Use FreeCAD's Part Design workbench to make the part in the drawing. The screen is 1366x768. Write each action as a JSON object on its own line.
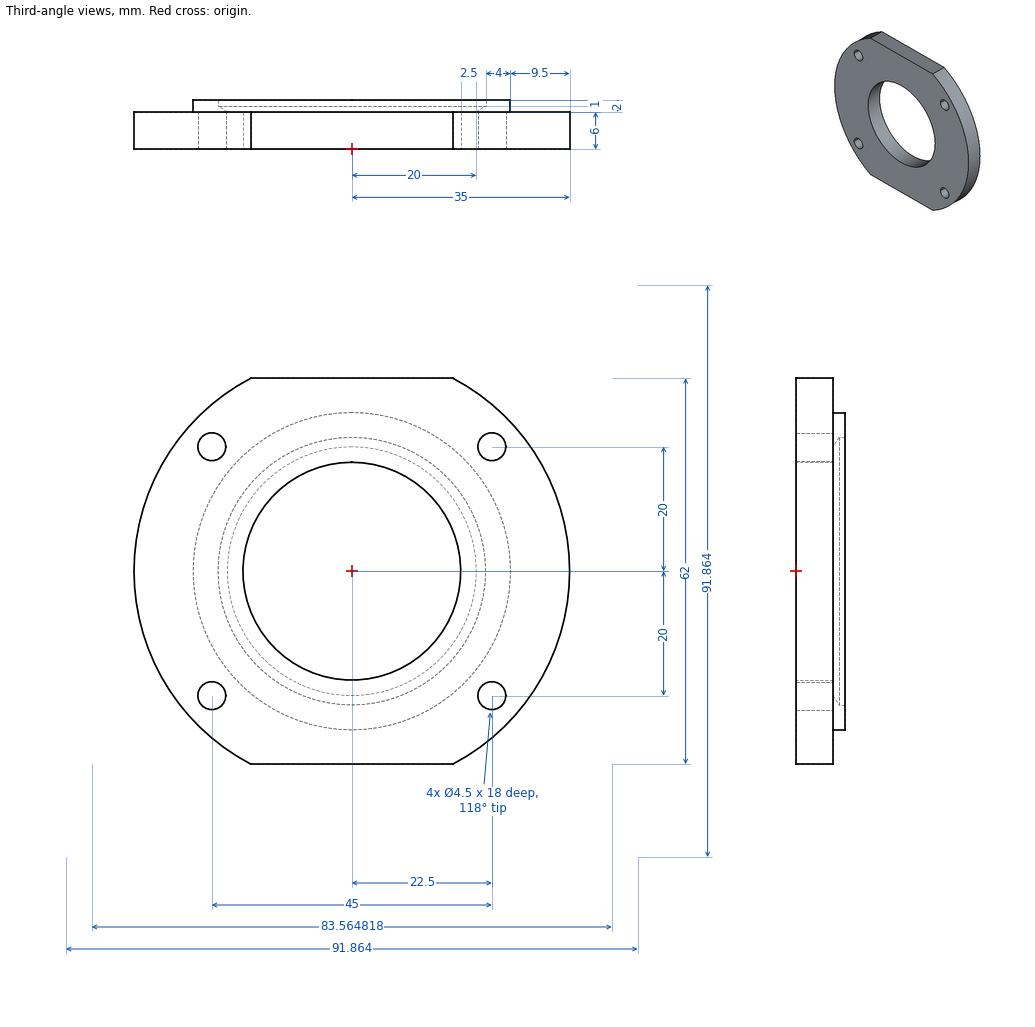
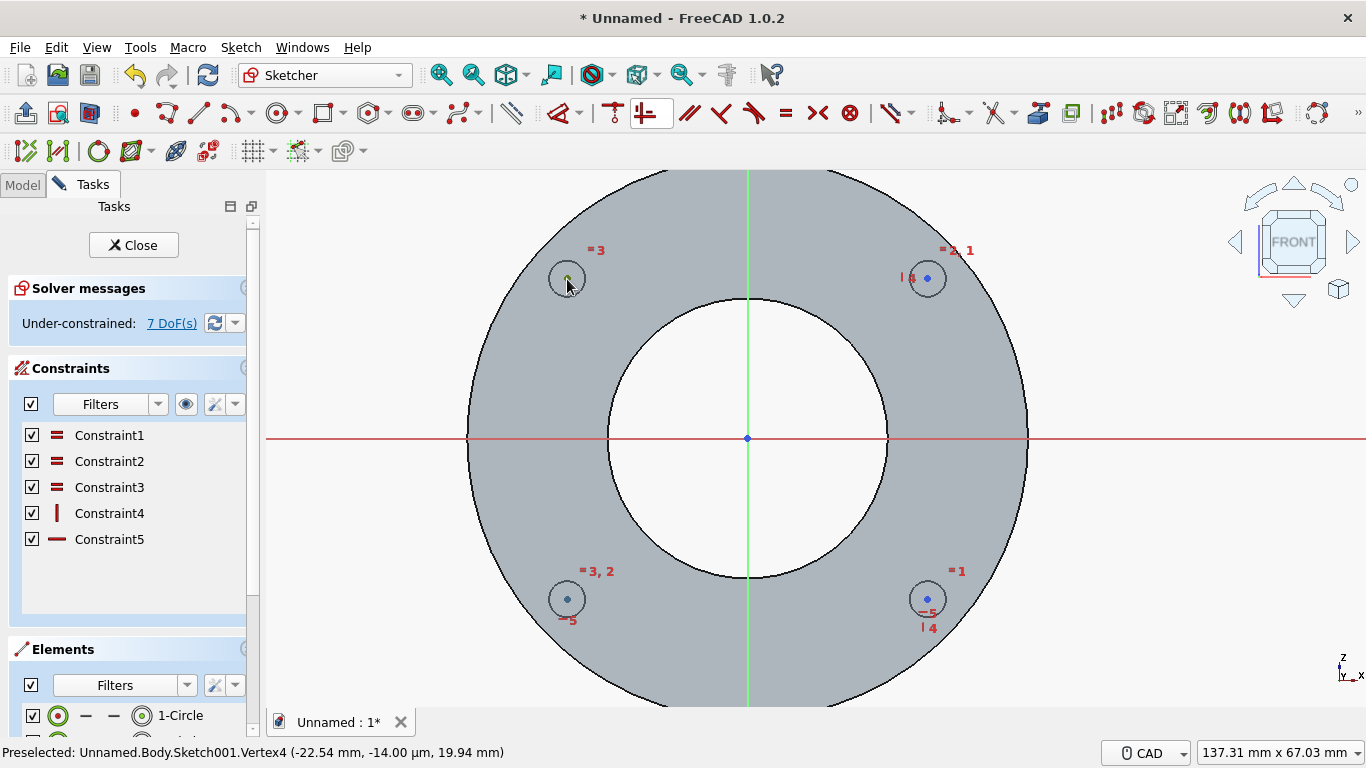
{"action": "key", "text": "v"}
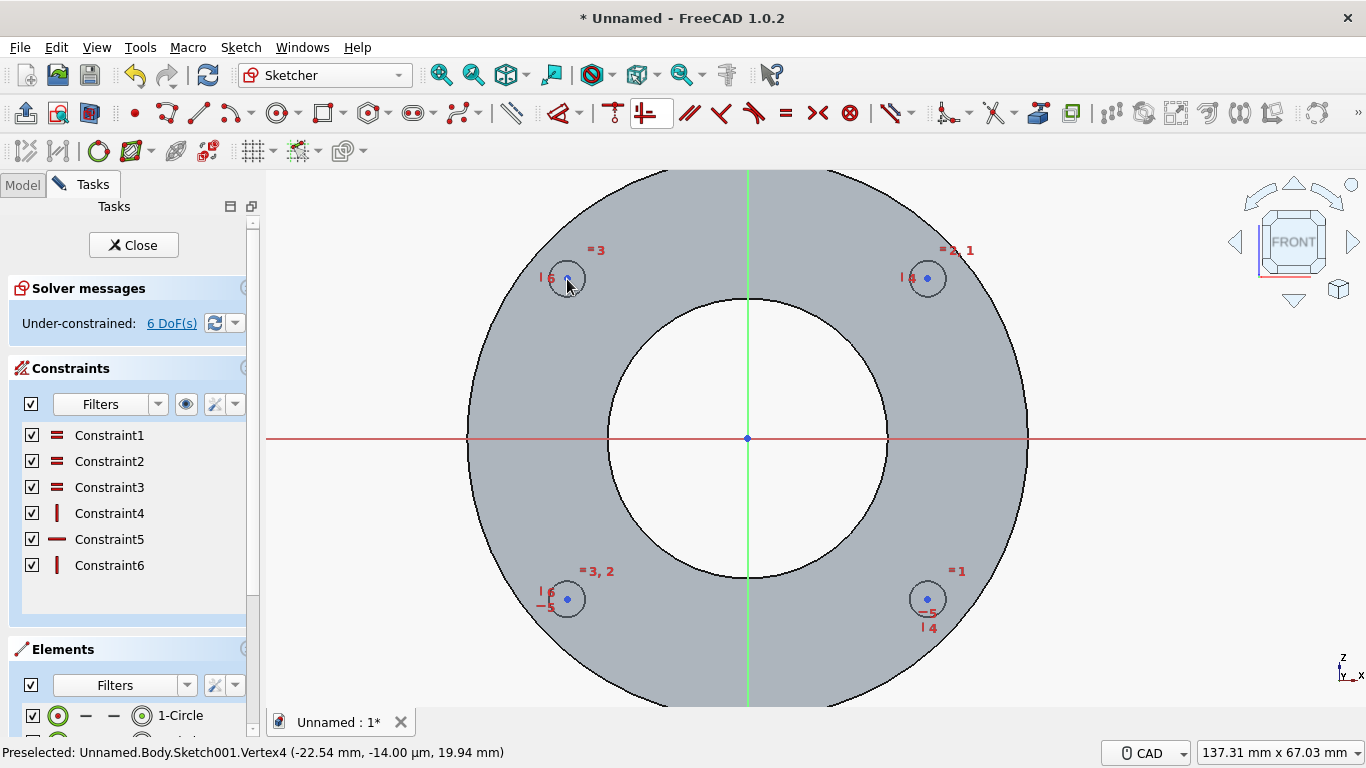
{"action": "left_click", "coordinate": [928, 279]}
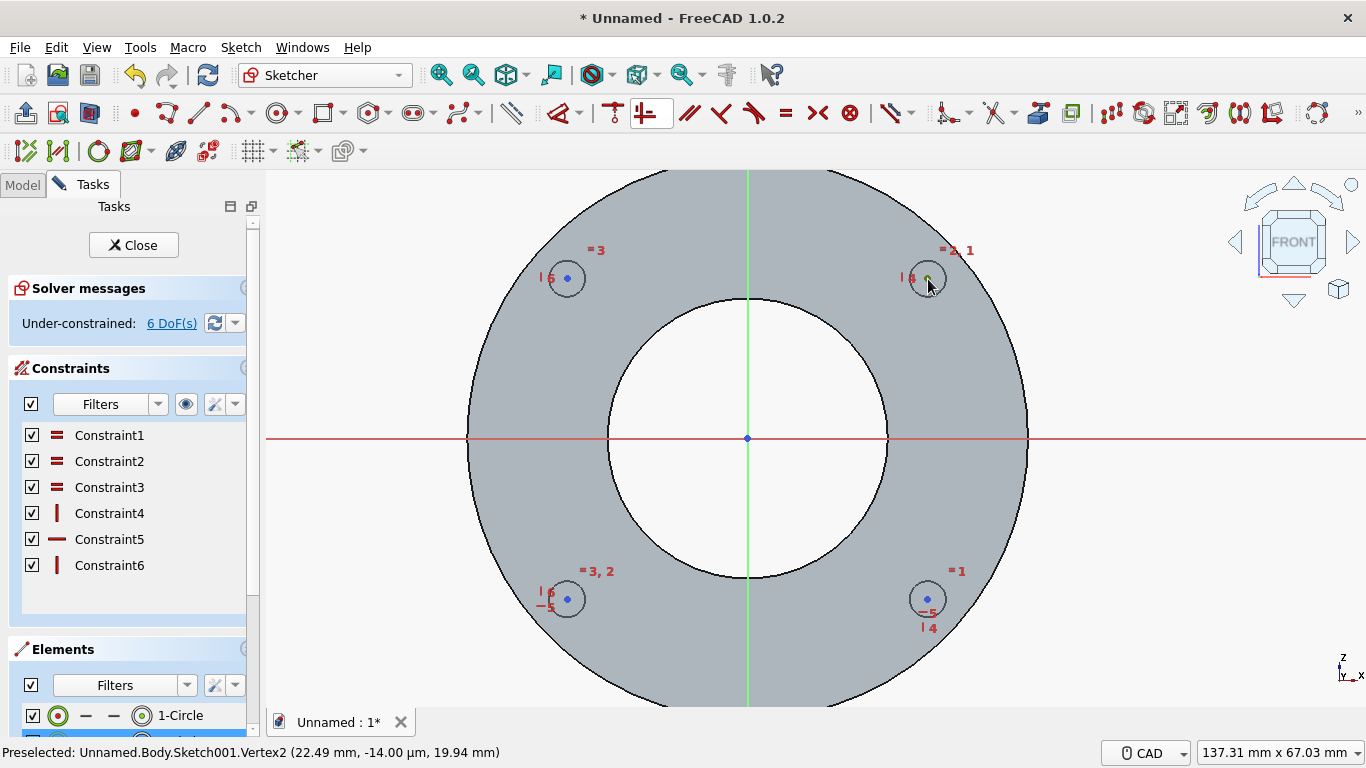
{"action": "left_click", "coordinate": [567, 279]}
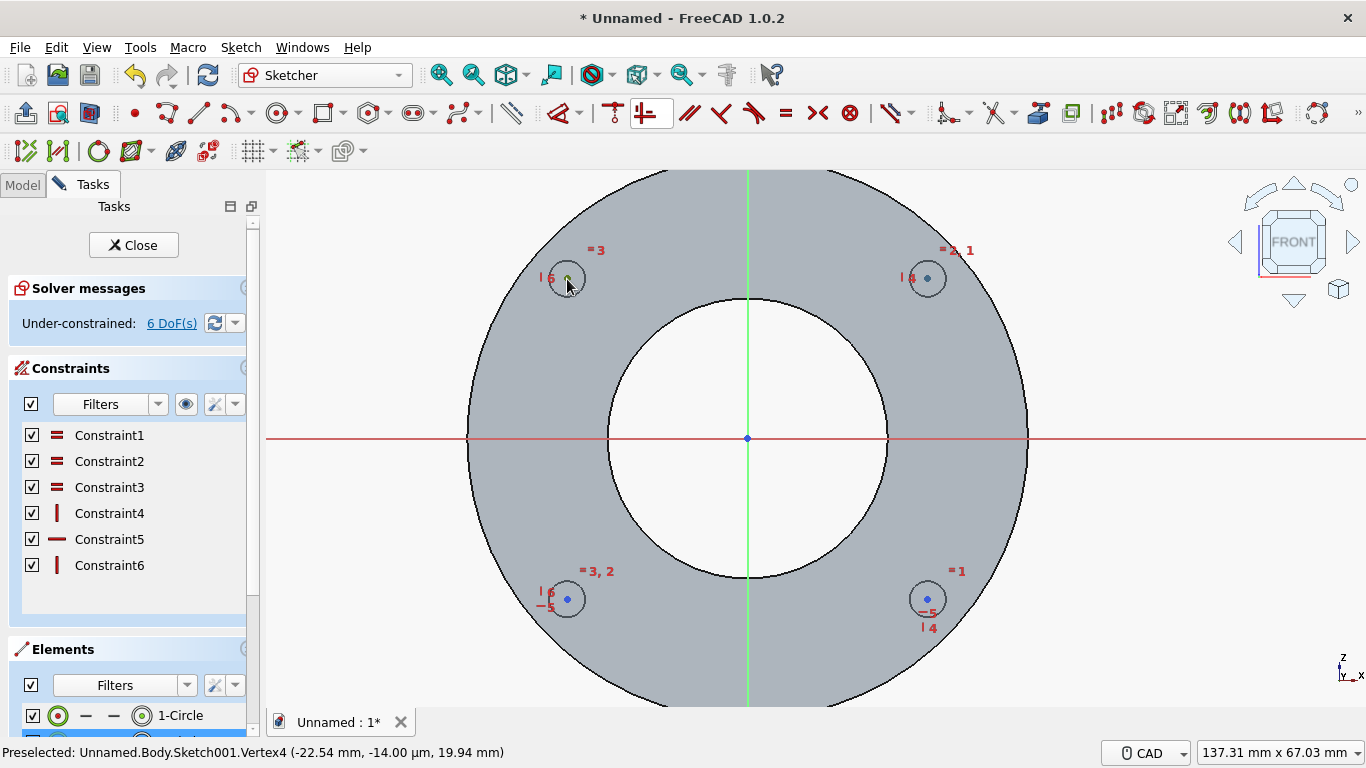
{"action": "key", "text": "h"}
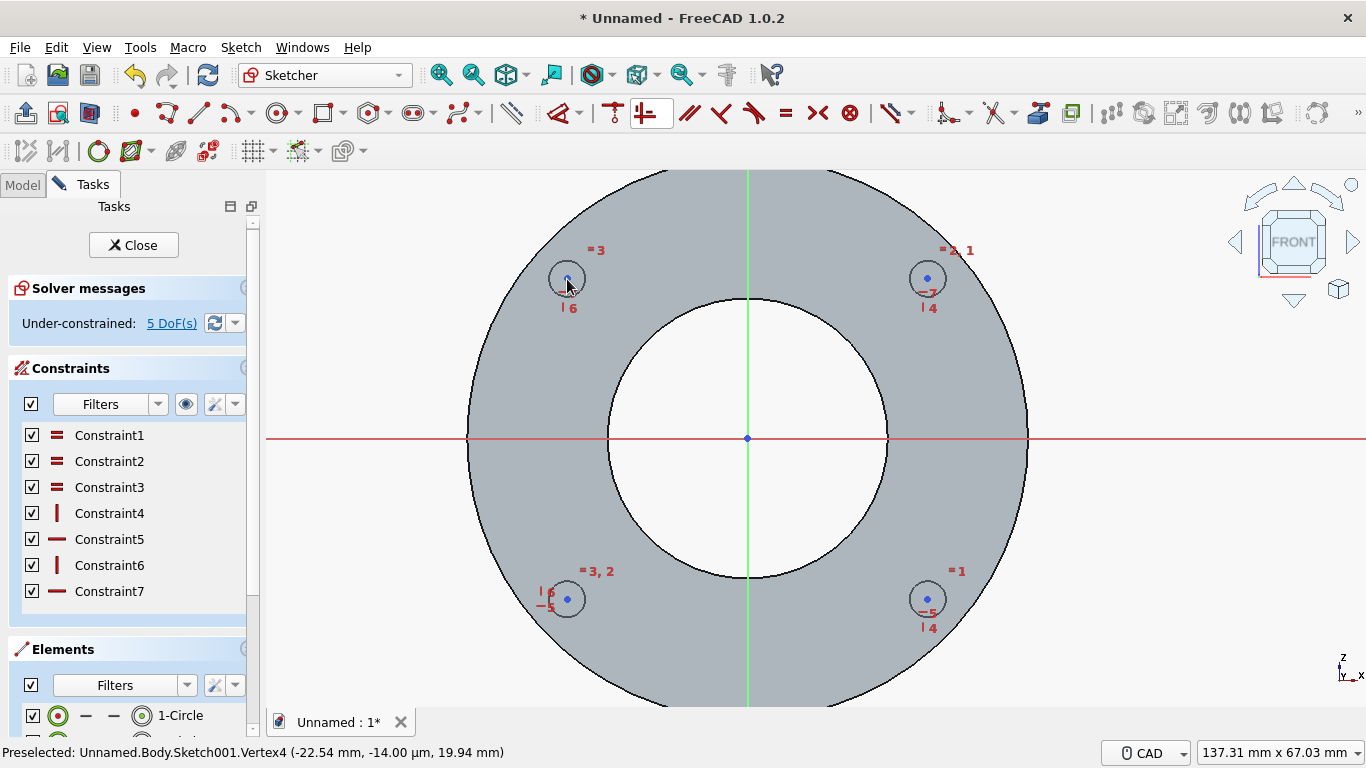
{"action": "left_click", "coordinate": [558, 114]}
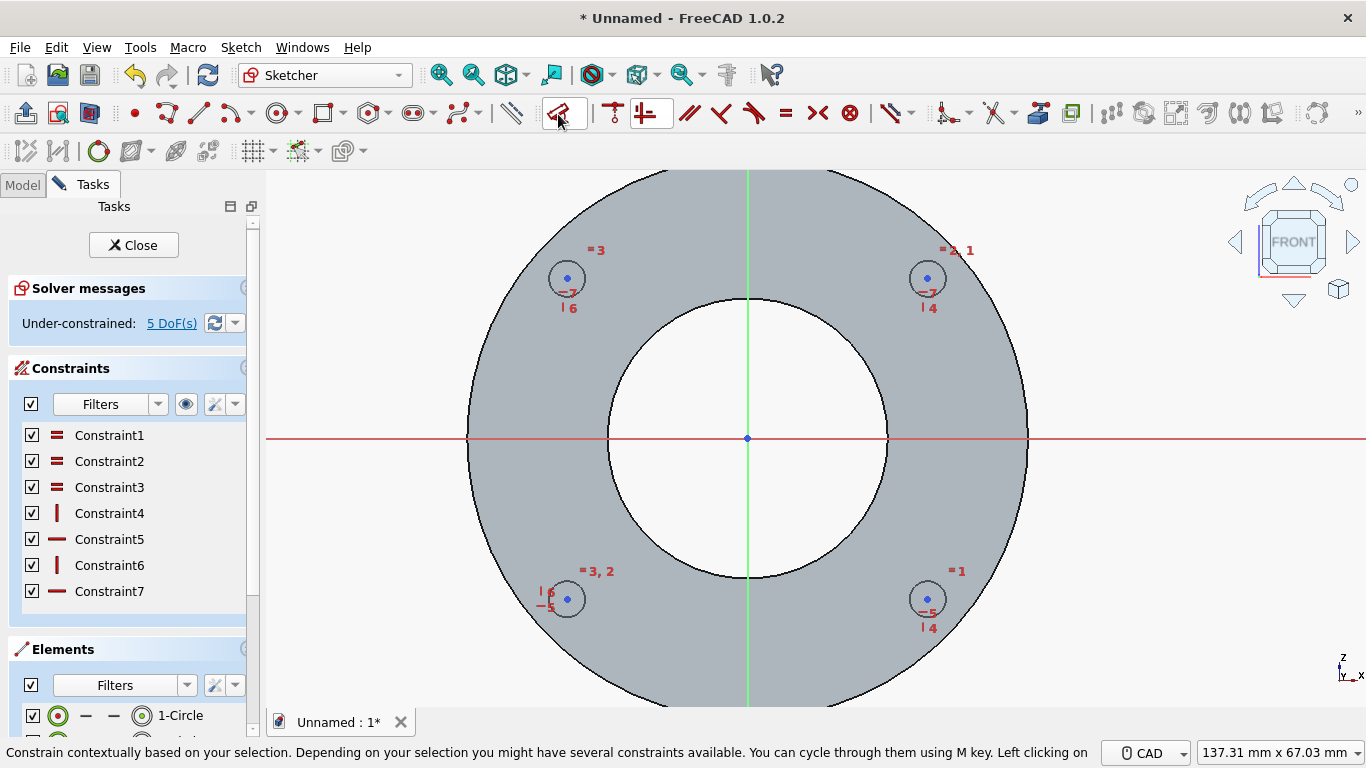
{"action": "left_click", "coordinate": [941, 586]}
{"action": "left_click", "coordinate": [964, 563]}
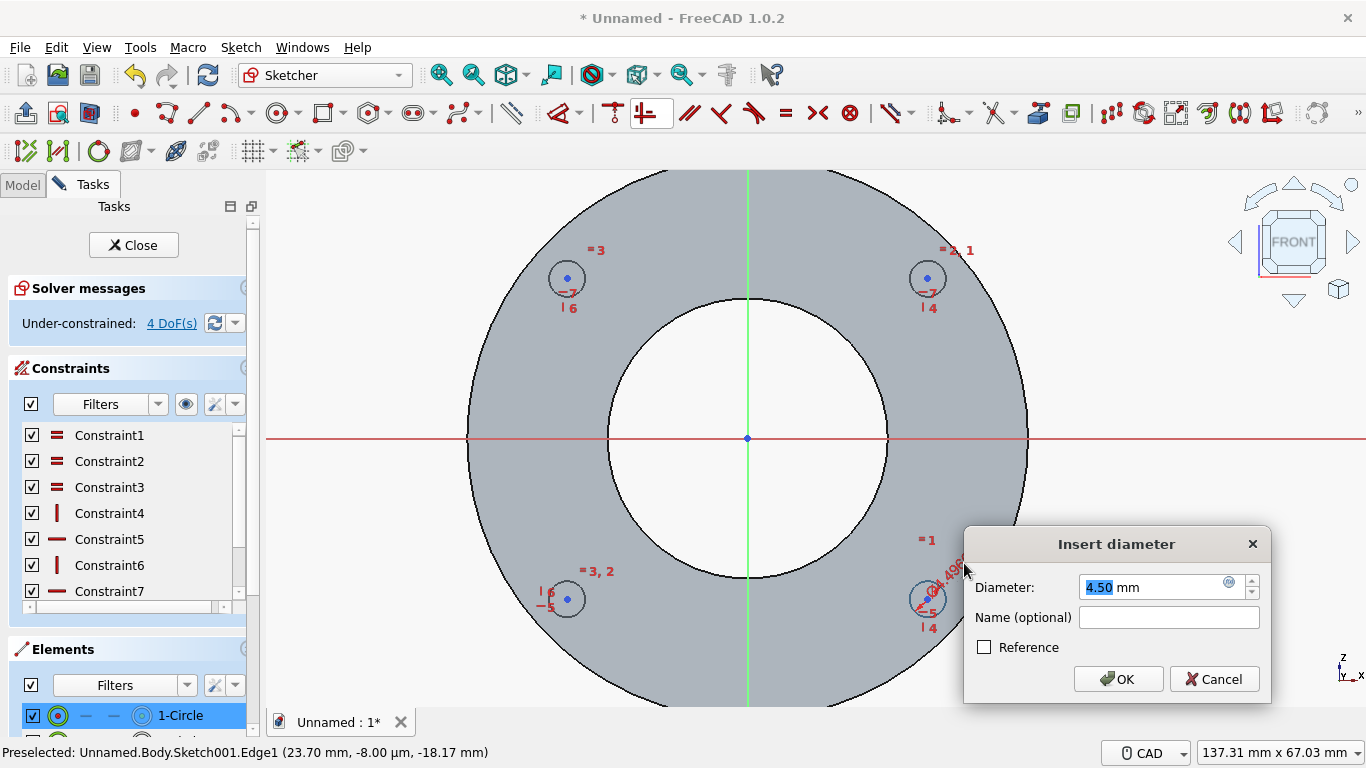
{"action": "type", "text": "4.5"}
{"action": "key", "text": "Return"}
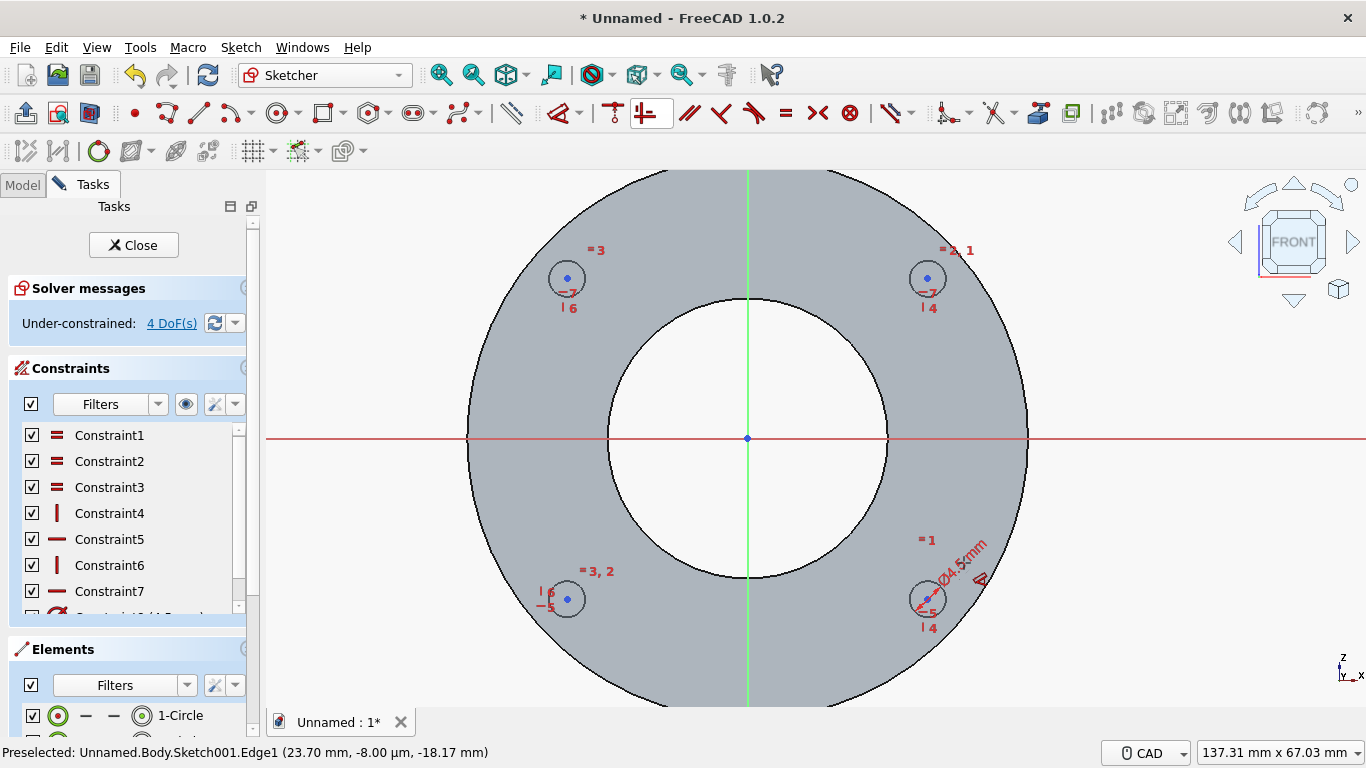
{"action": "left_click", "coordinate": [928, 599]}
{"action": "left_click", "coordinate": [962, 519]}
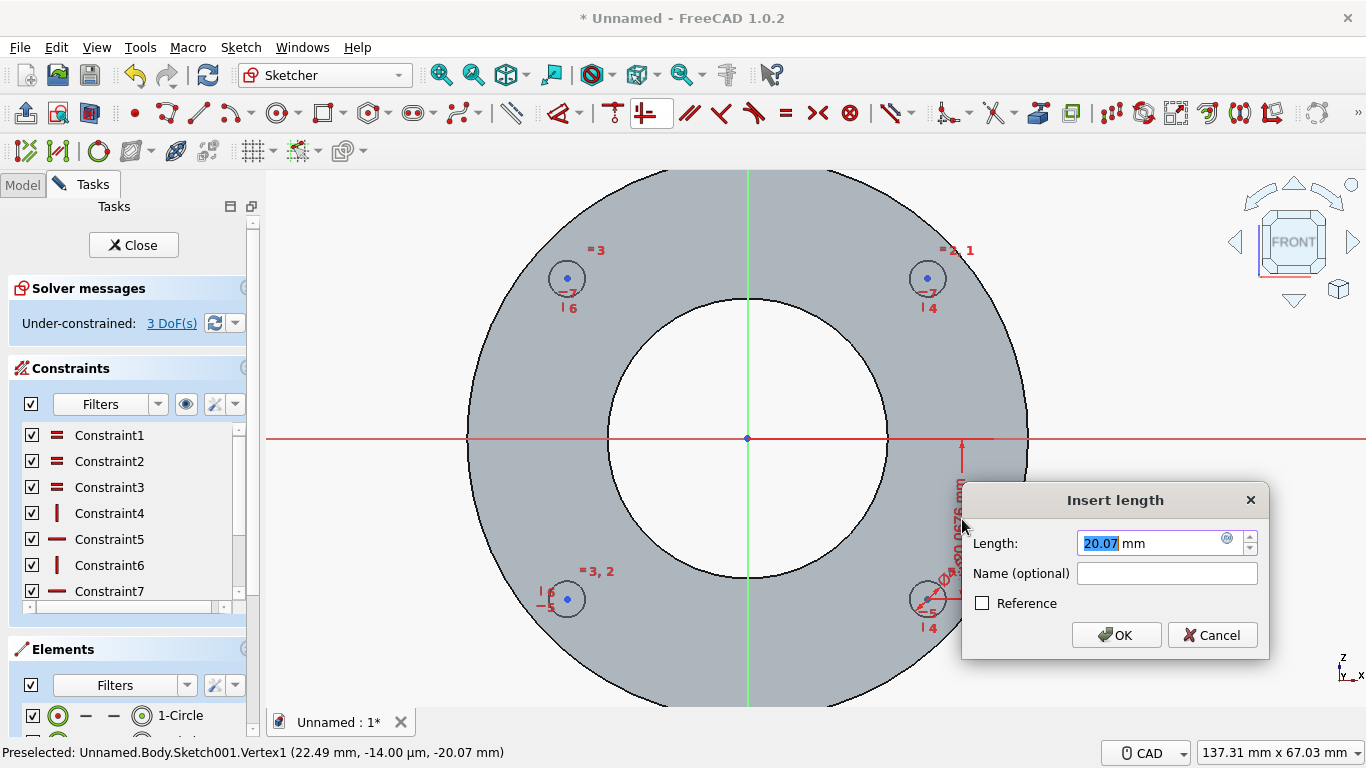
{"action": "type", "text": "20"}
{"action": "key", "text": "Return"}